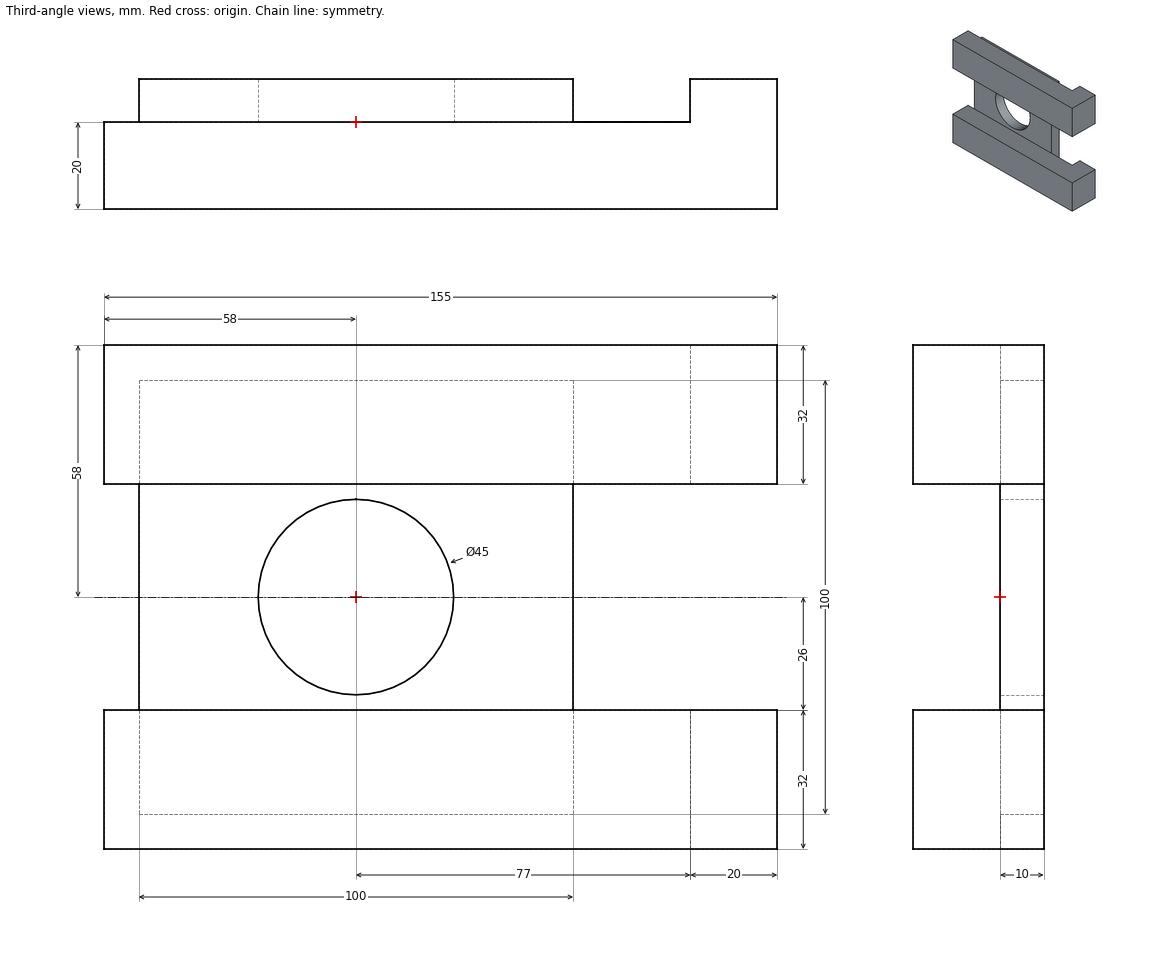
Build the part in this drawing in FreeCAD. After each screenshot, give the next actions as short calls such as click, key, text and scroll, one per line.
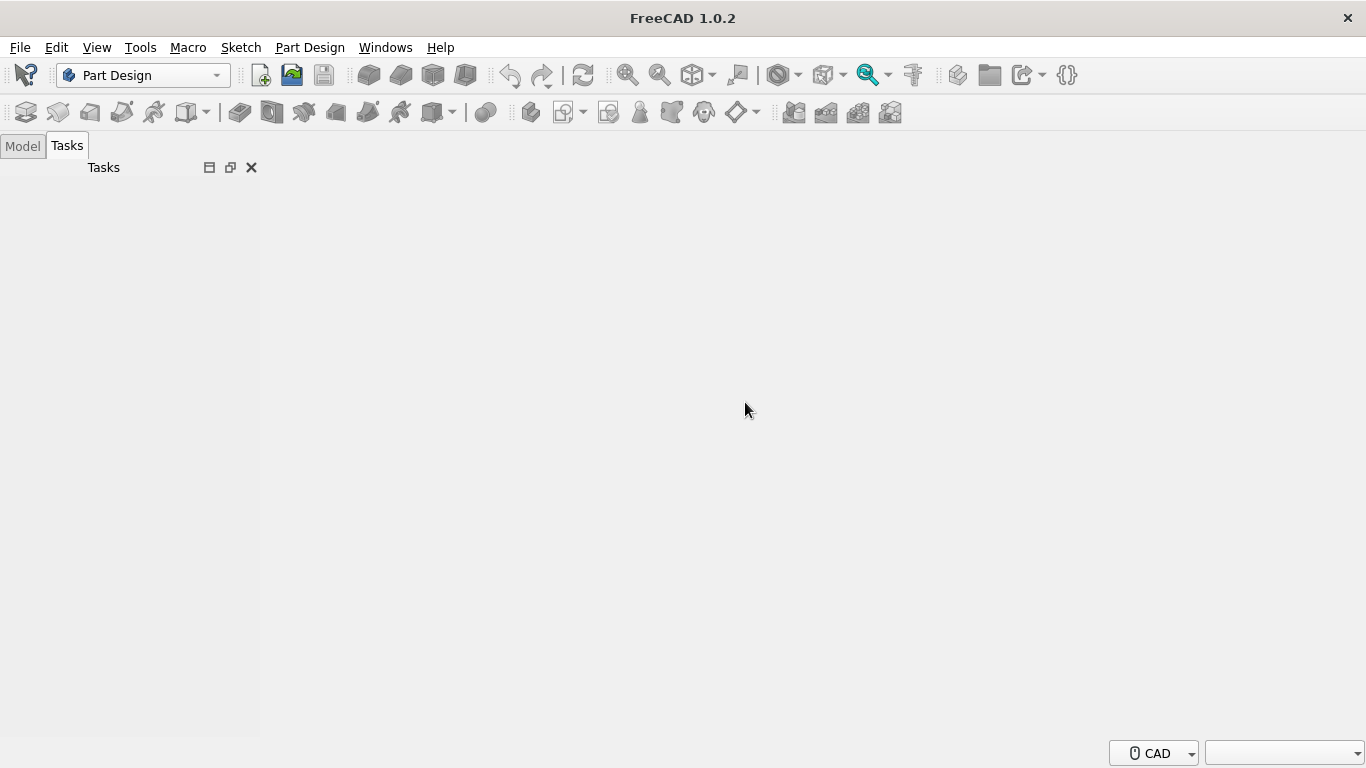
key(ctrl+n)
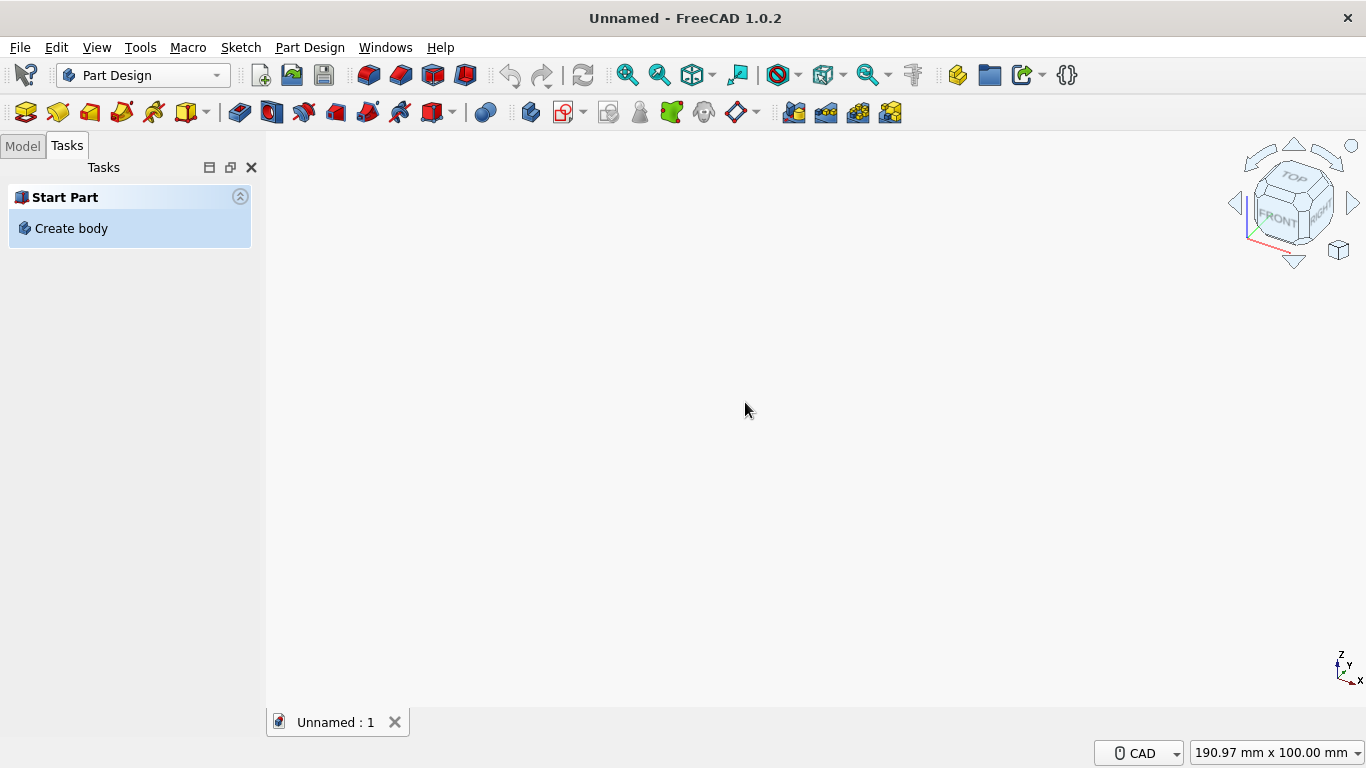
click(564, 112)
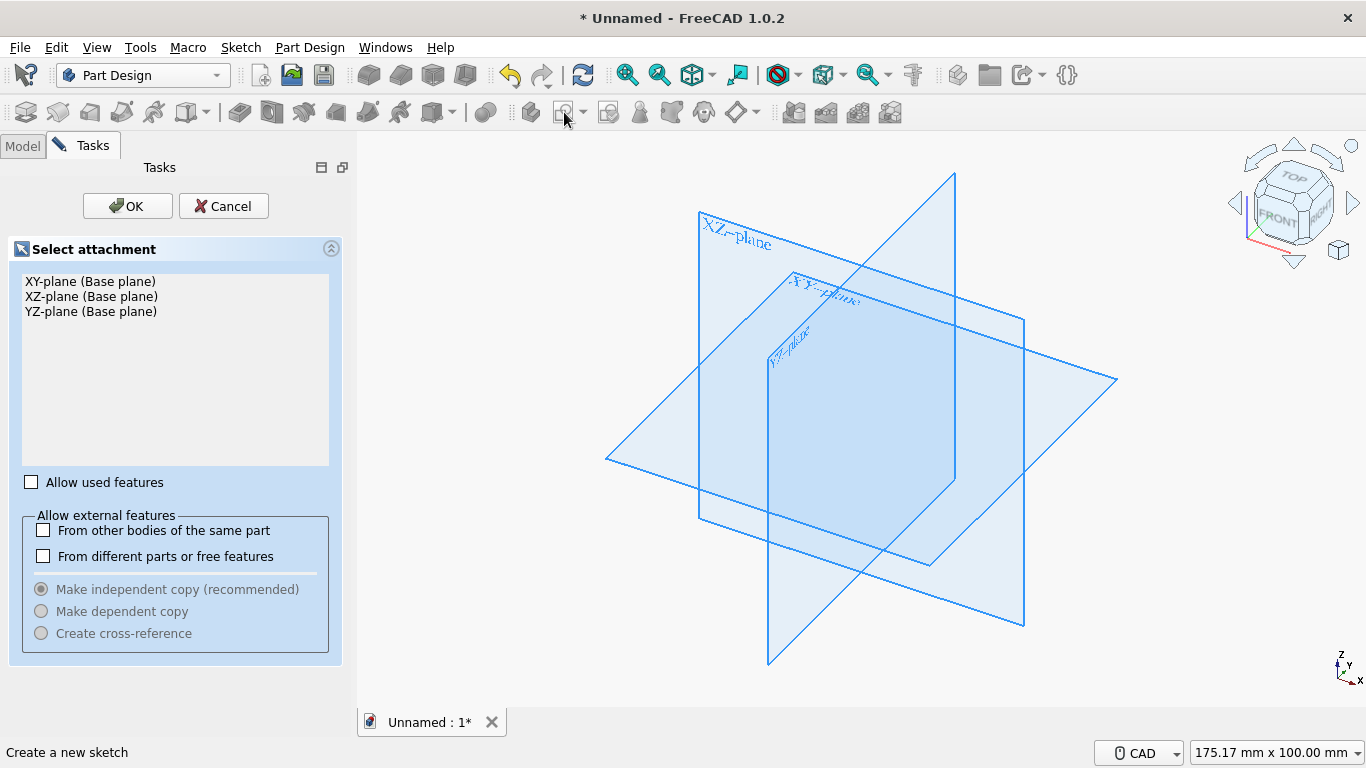
click(82, 296)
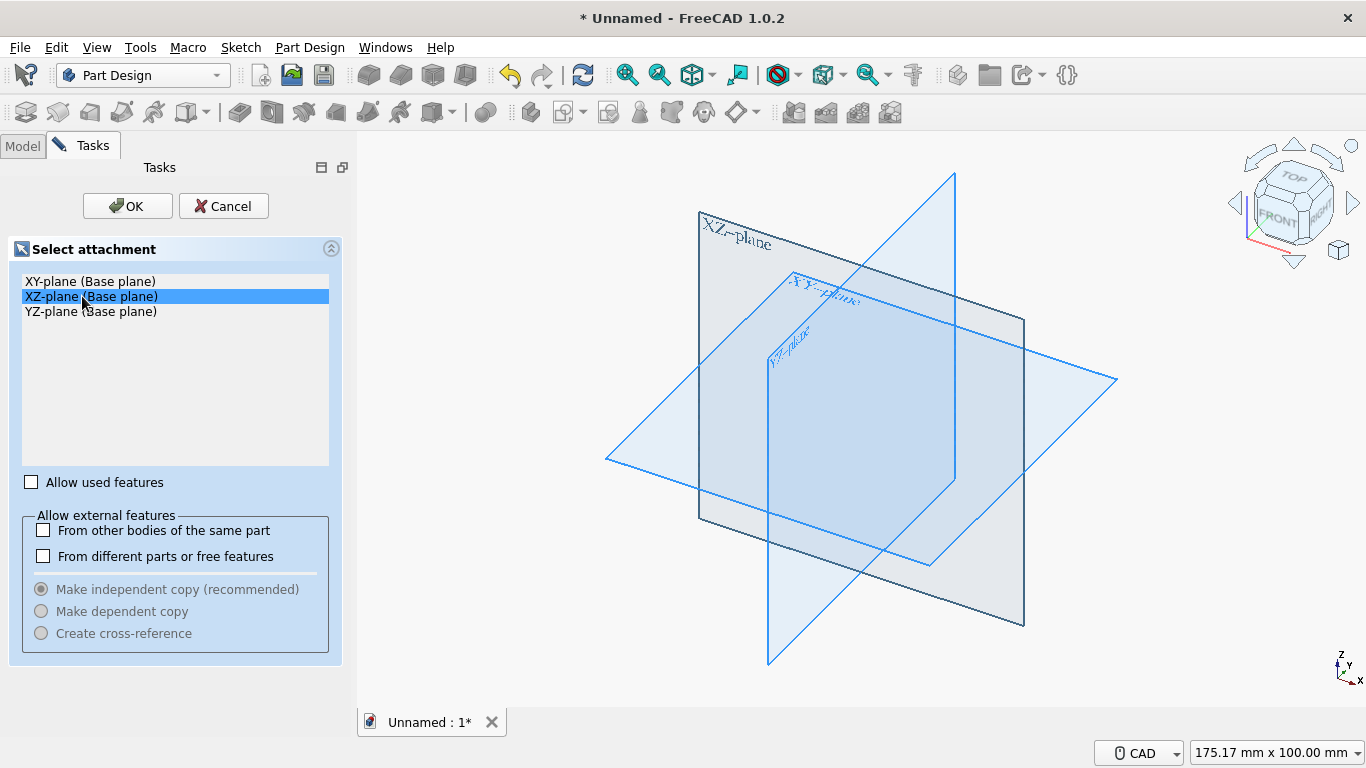
click(128, 206)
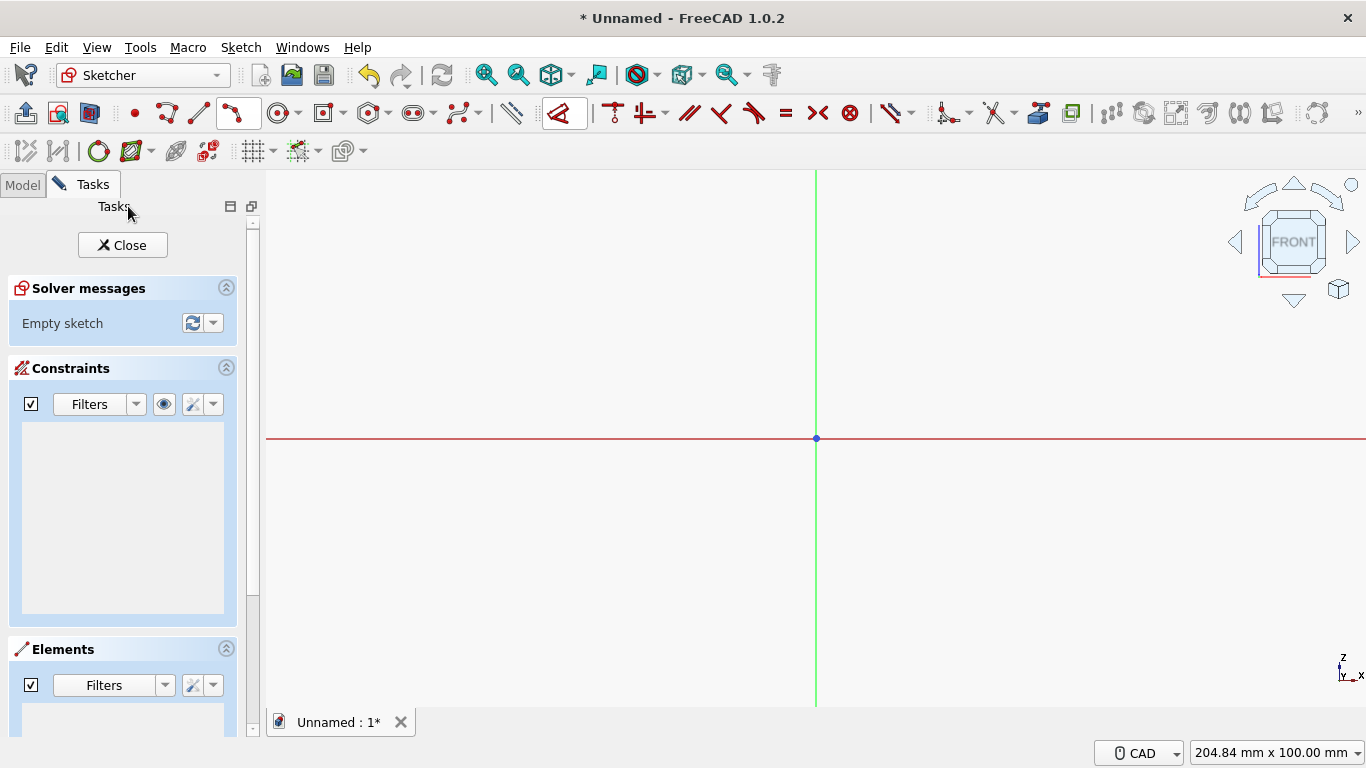
scroll(608, 438, down, 2)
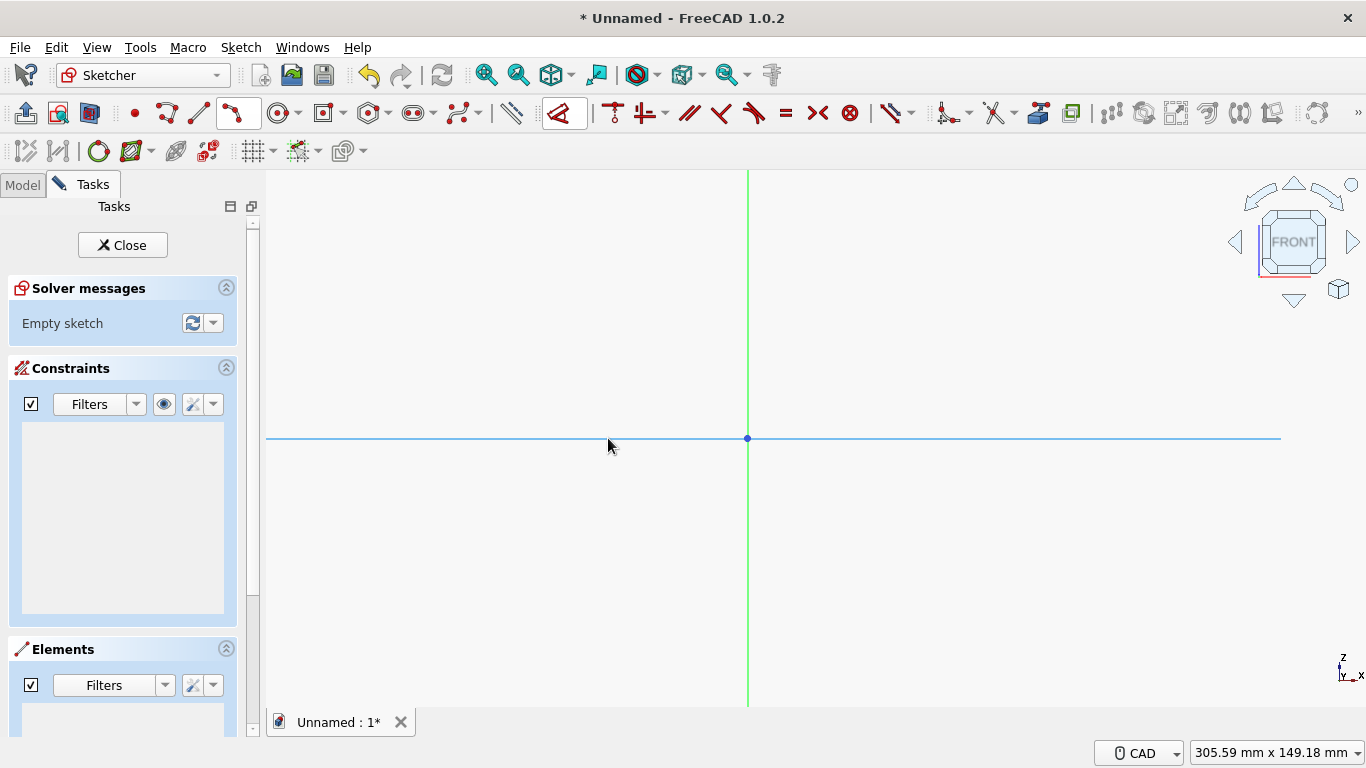
key(g)
key(v)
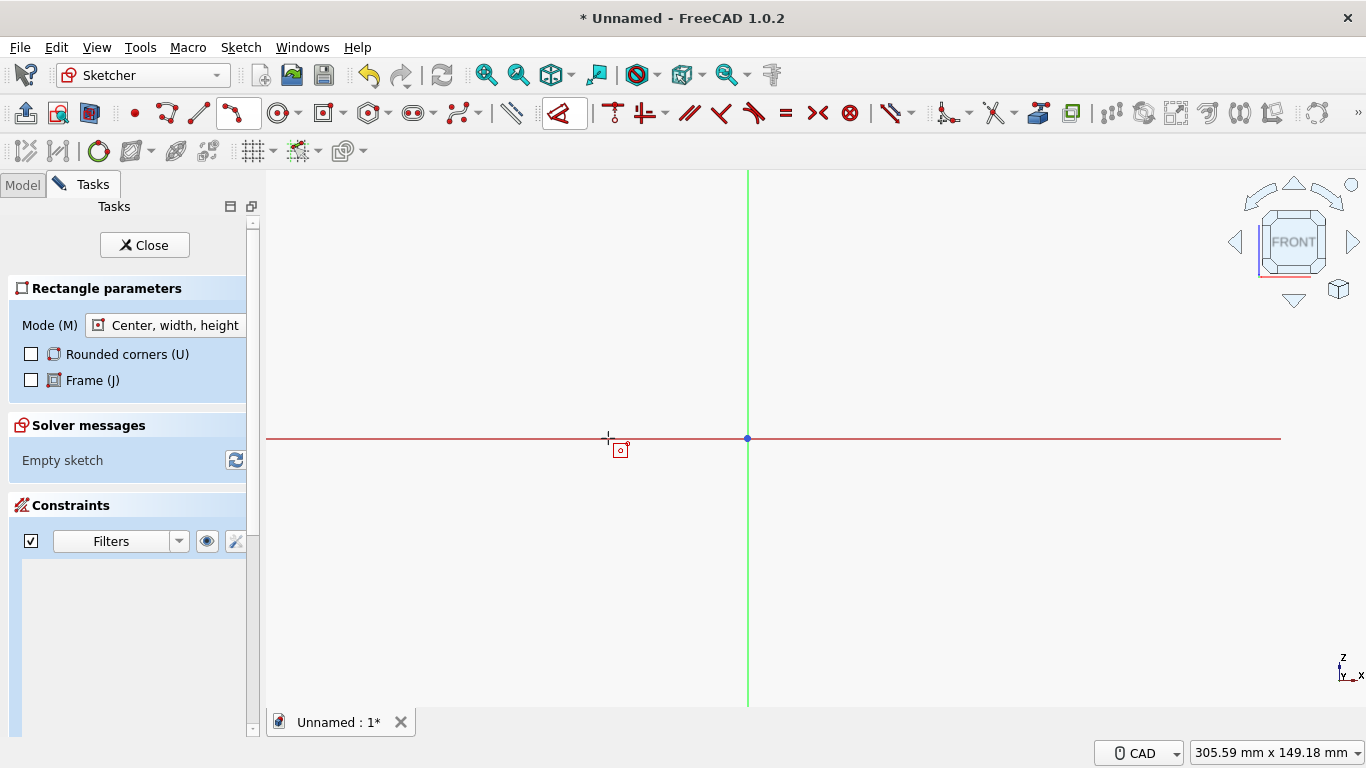
click(748, 438)
move(928, 259)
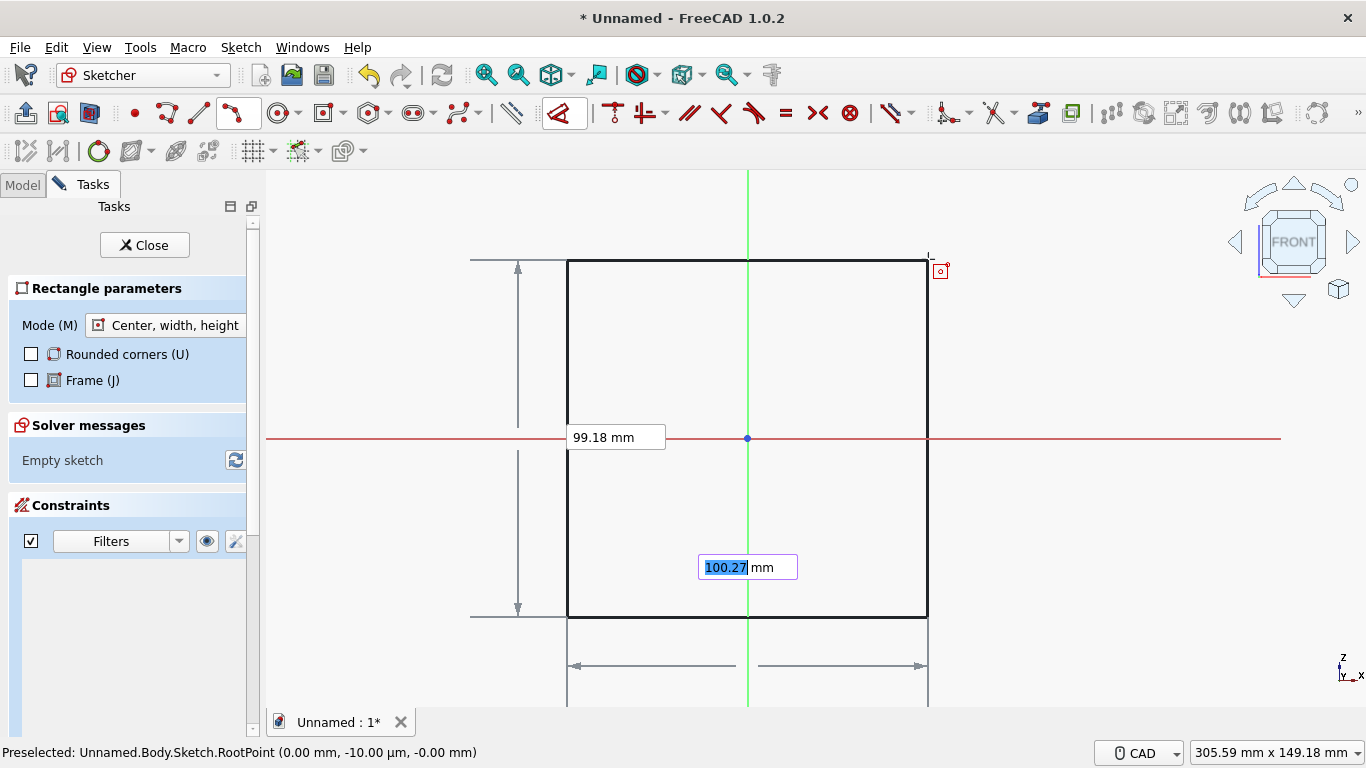
text(100)
key(Tab)
text(100)
key(Return)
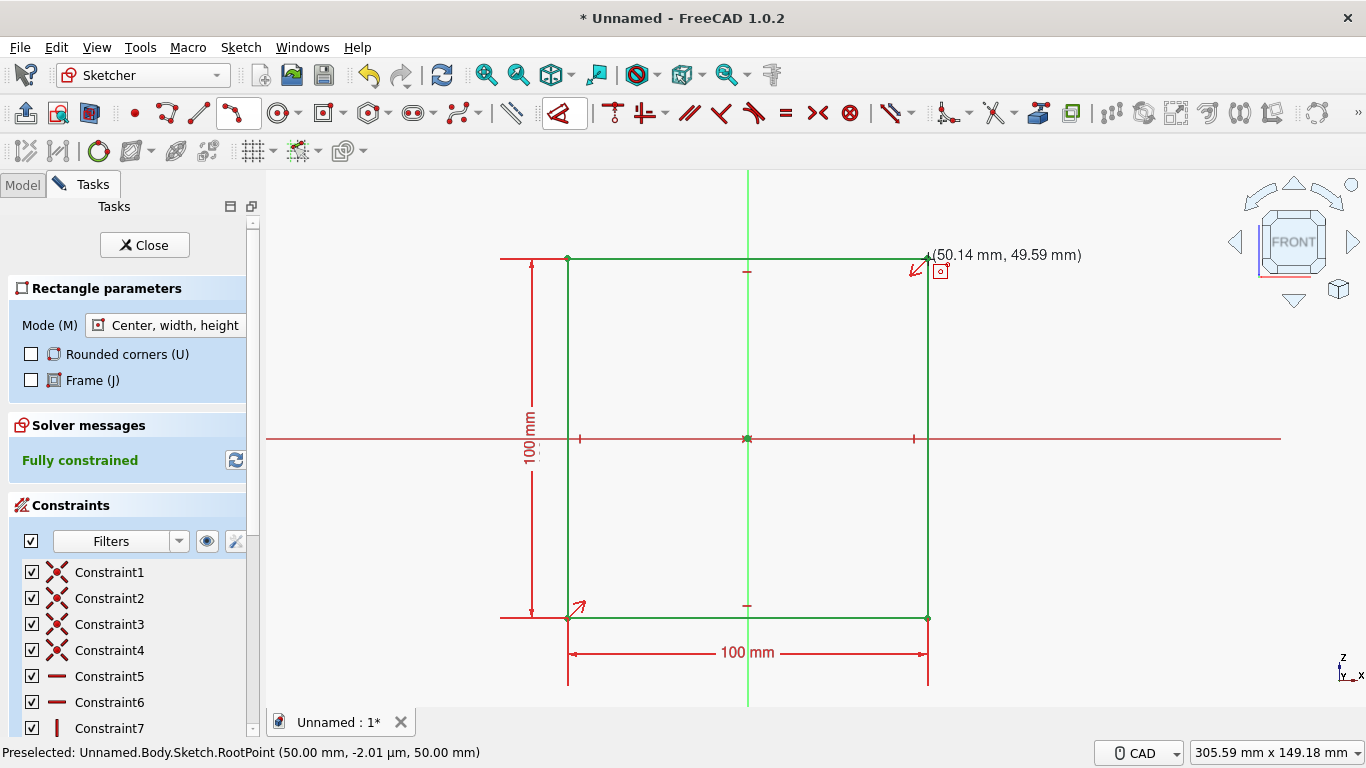
click(278, 114)